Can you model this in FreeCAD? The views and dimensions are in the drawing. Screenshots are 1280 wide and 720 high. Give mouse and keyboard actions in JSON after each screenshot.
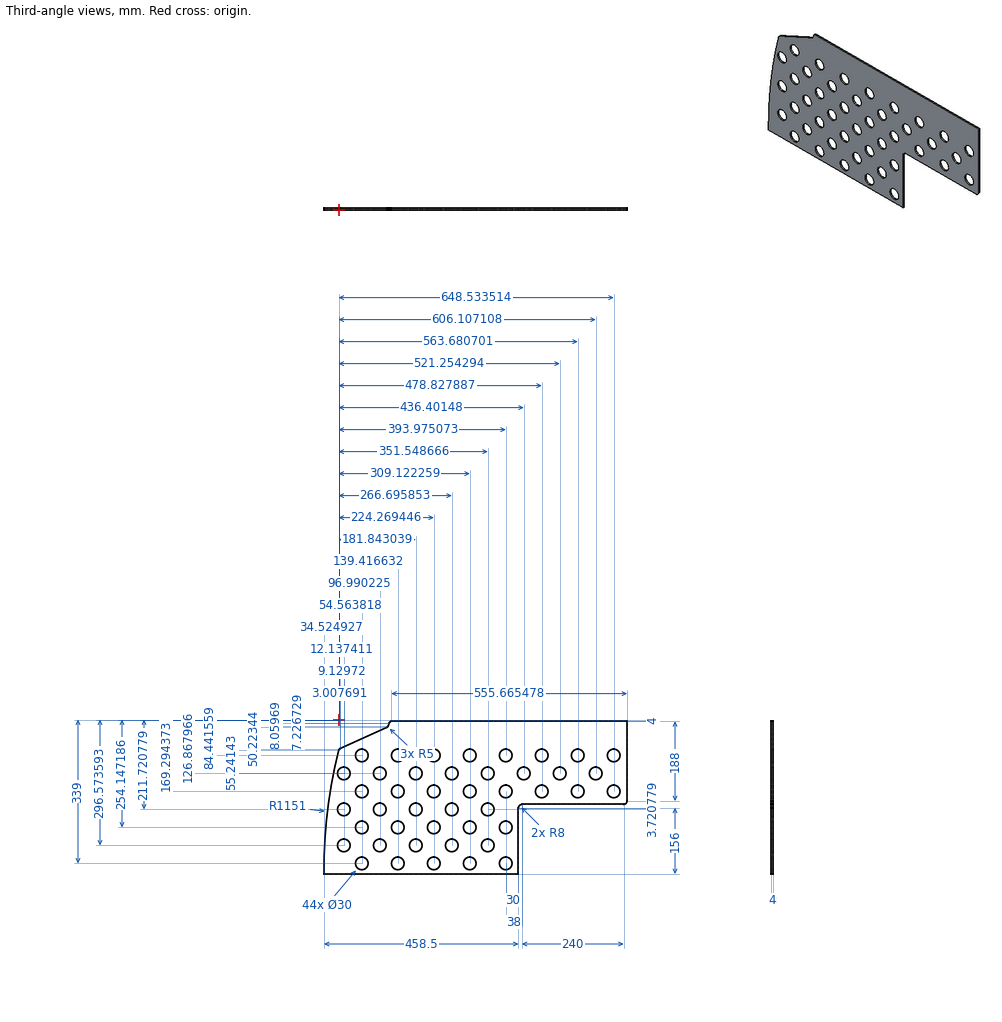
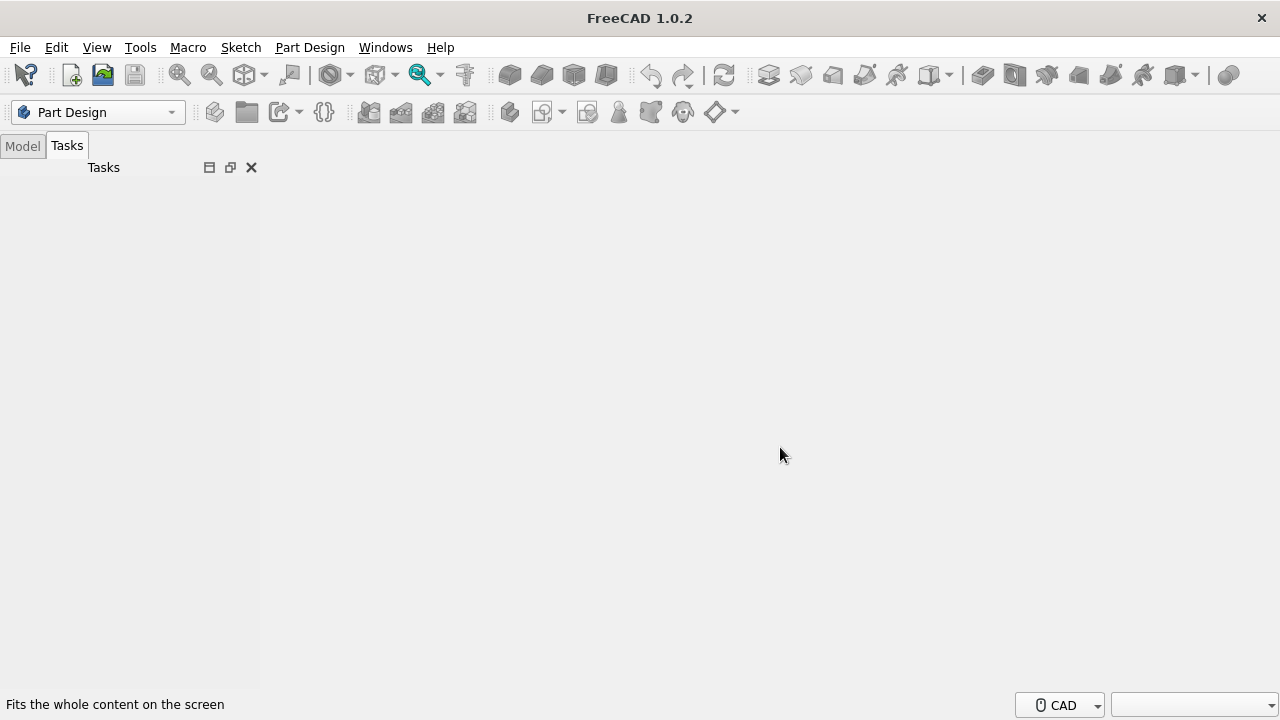
{"action": "key", "text": "ctrl+n"}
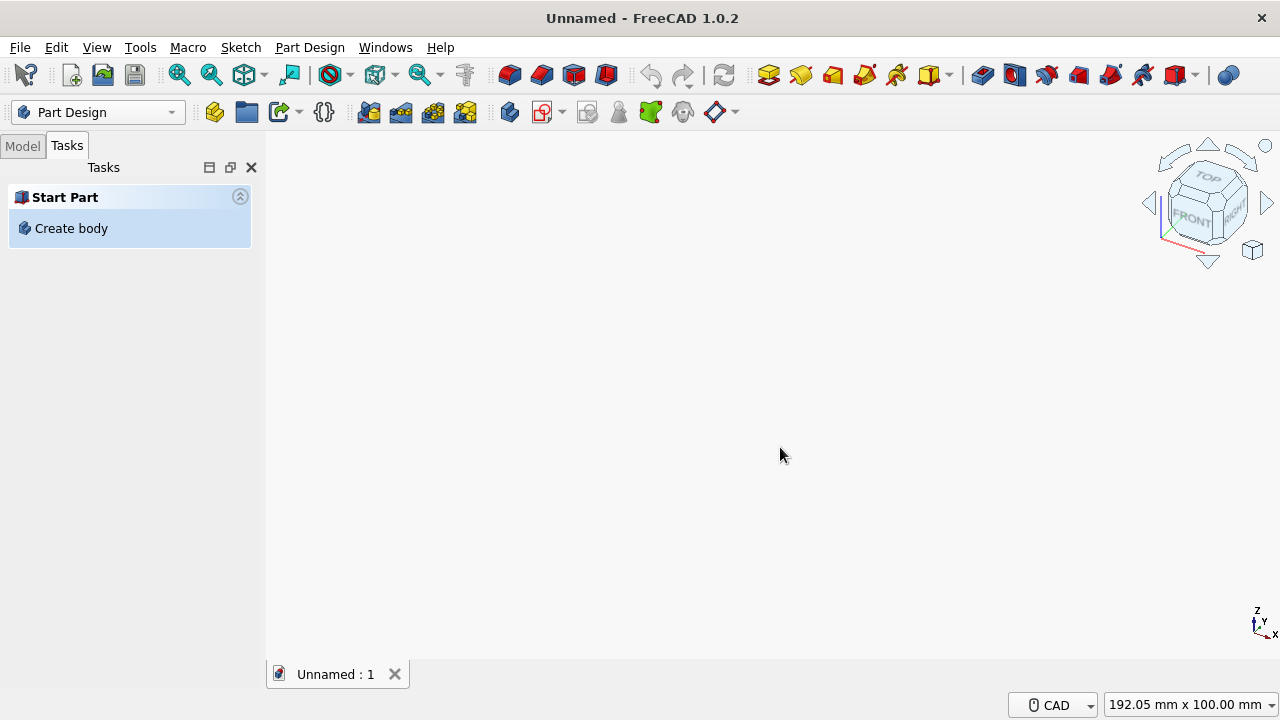
{"action": "left_click", "coordinate": [542, 112]}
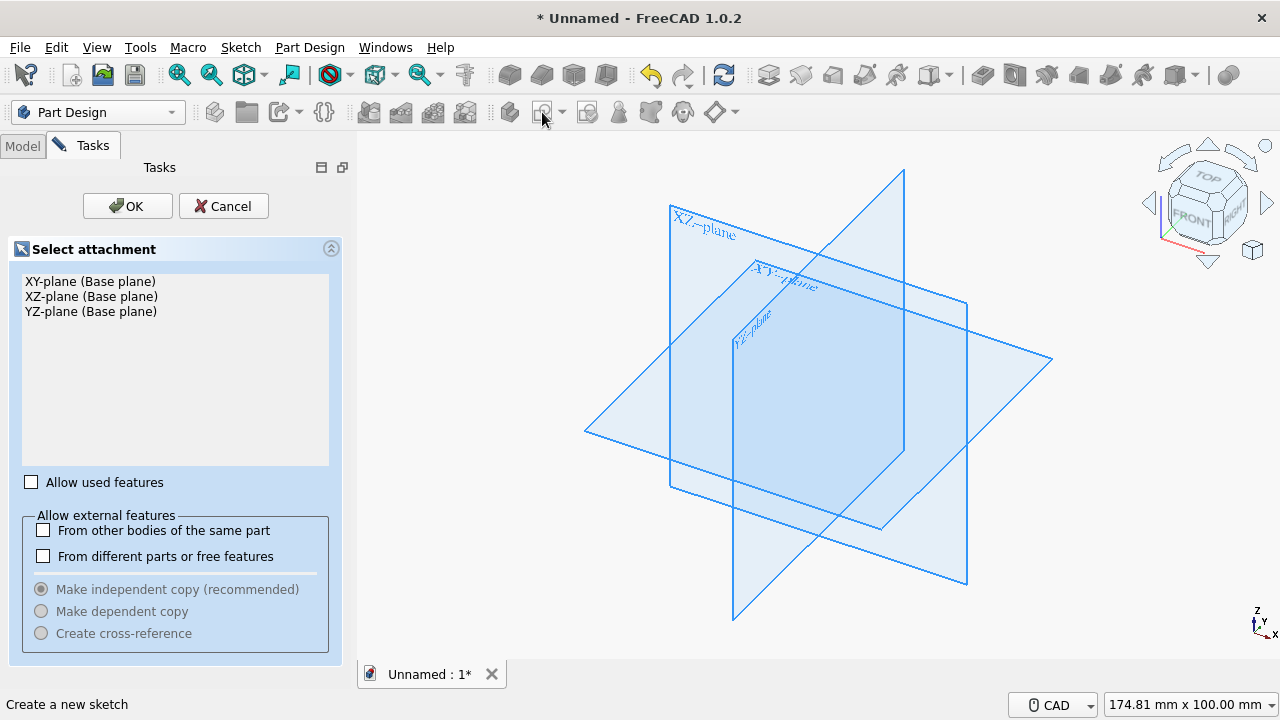
{"action": "left_click", "coordinate": [82, 296]}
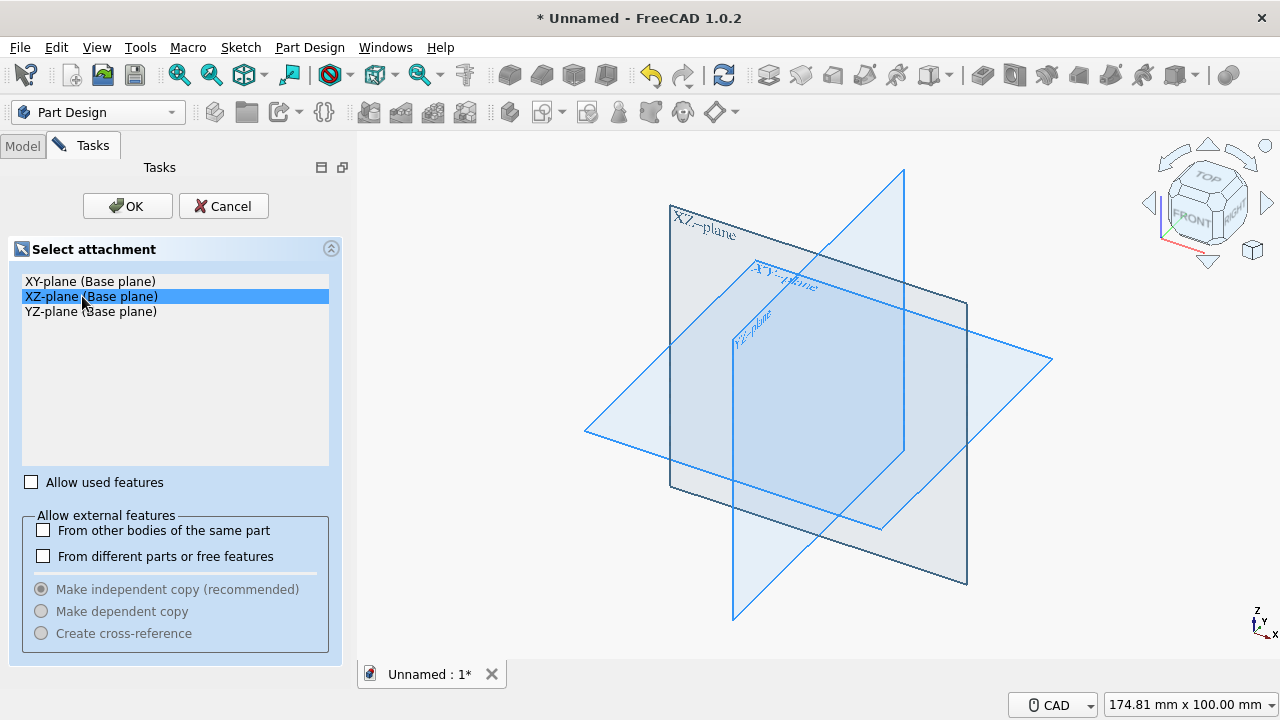
{"action": "left_click", "coordinate": [128, 206]}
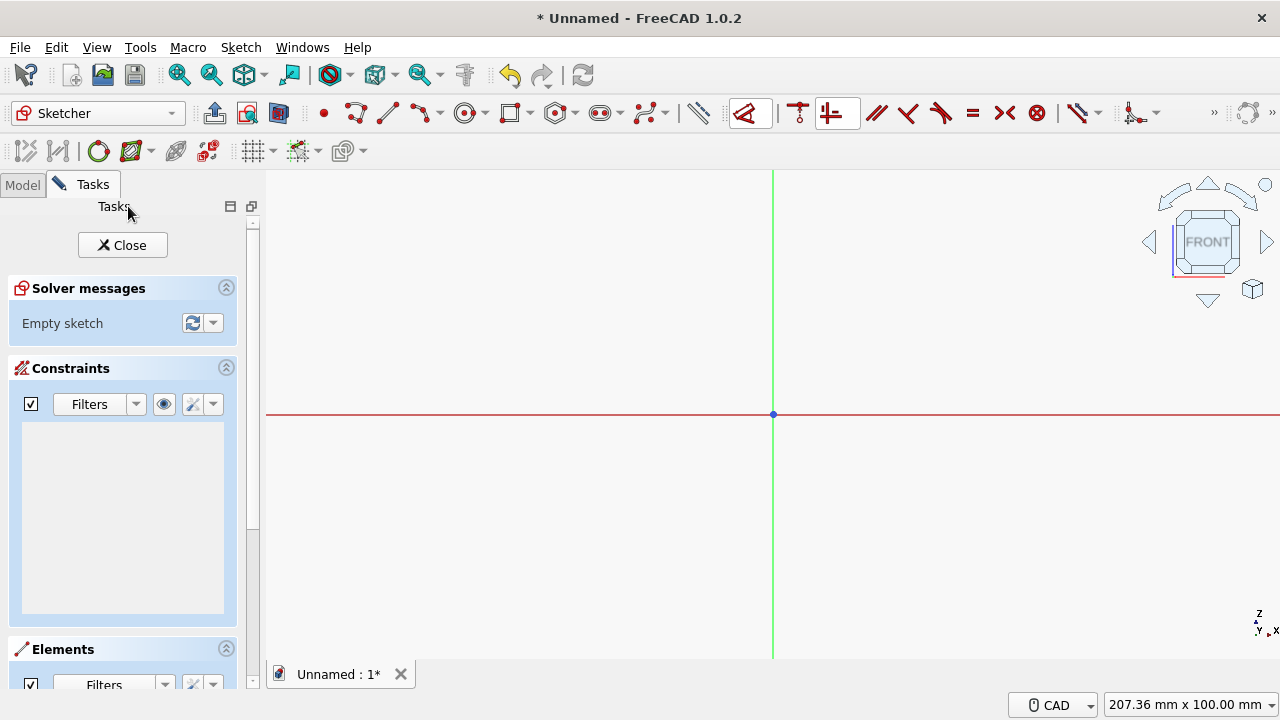
{"action": "scroll", "coordinate": [378, 238], "scroll_direction": "down", "scroll_amount": 9}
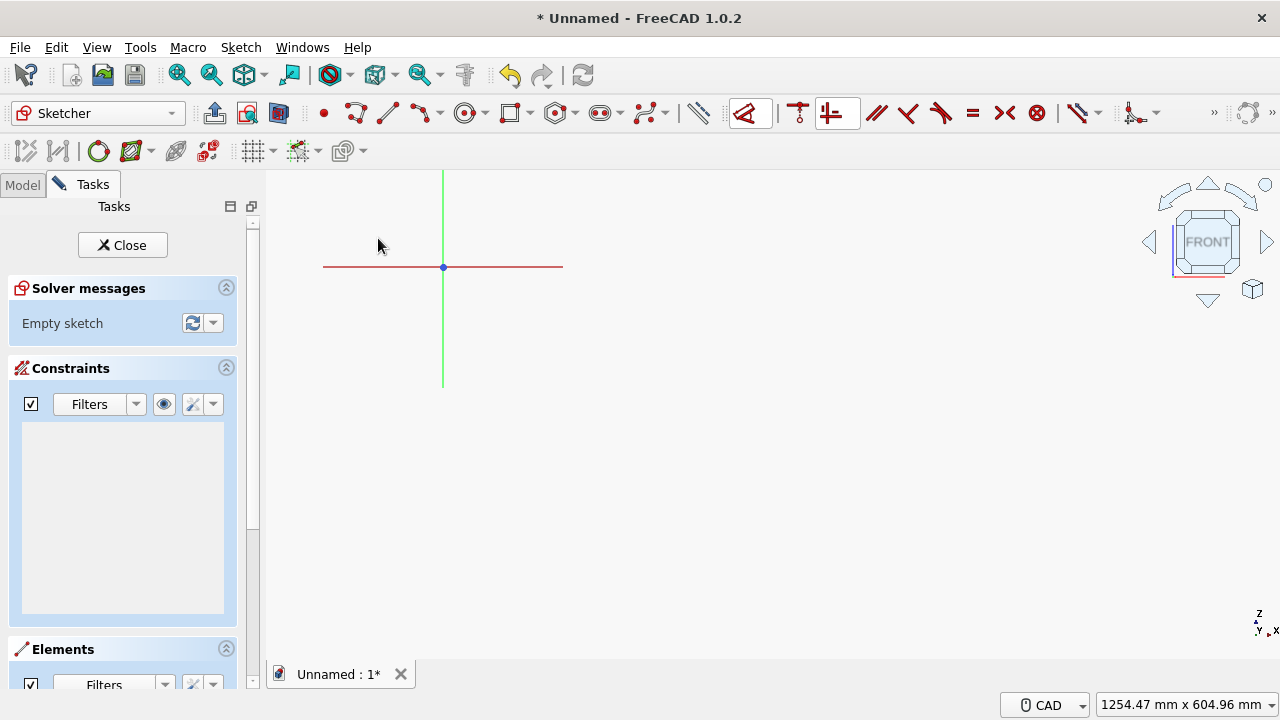
{"action": "key", "text": "g l"}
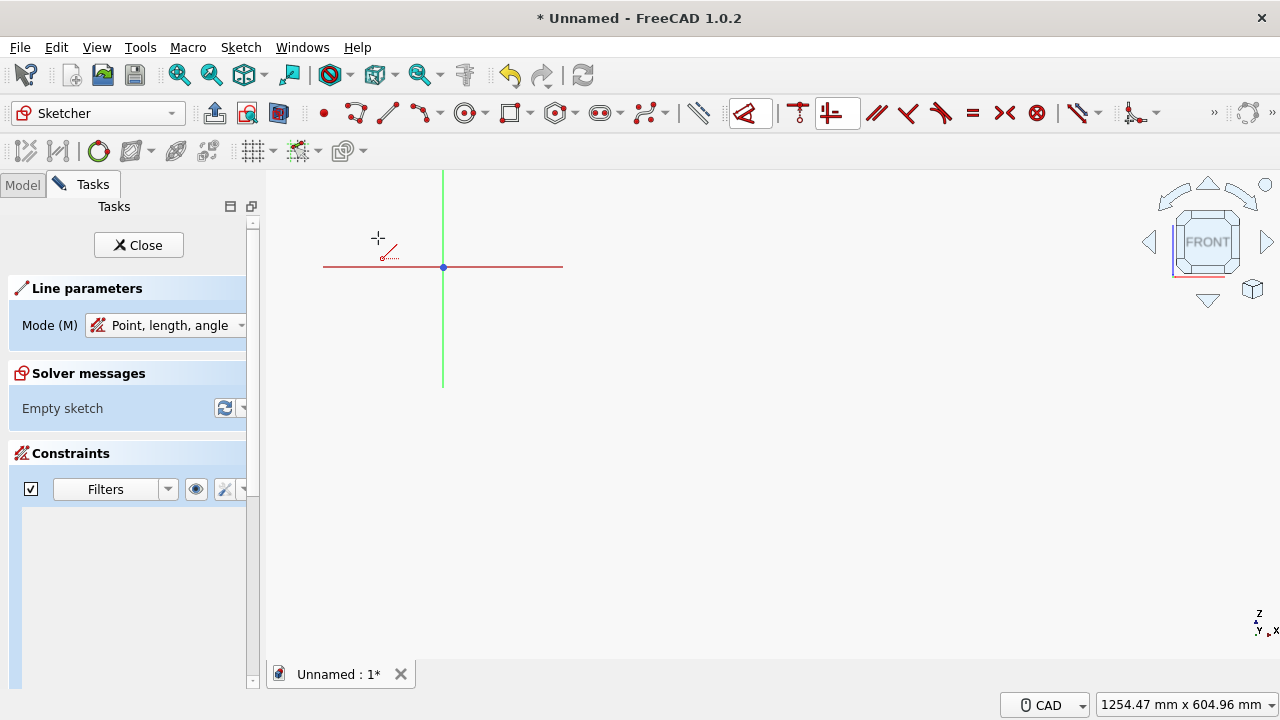
{"action": "scroll", "coordinate": [540, 273], "scroll_direction": "up", "scroll_amount": 5}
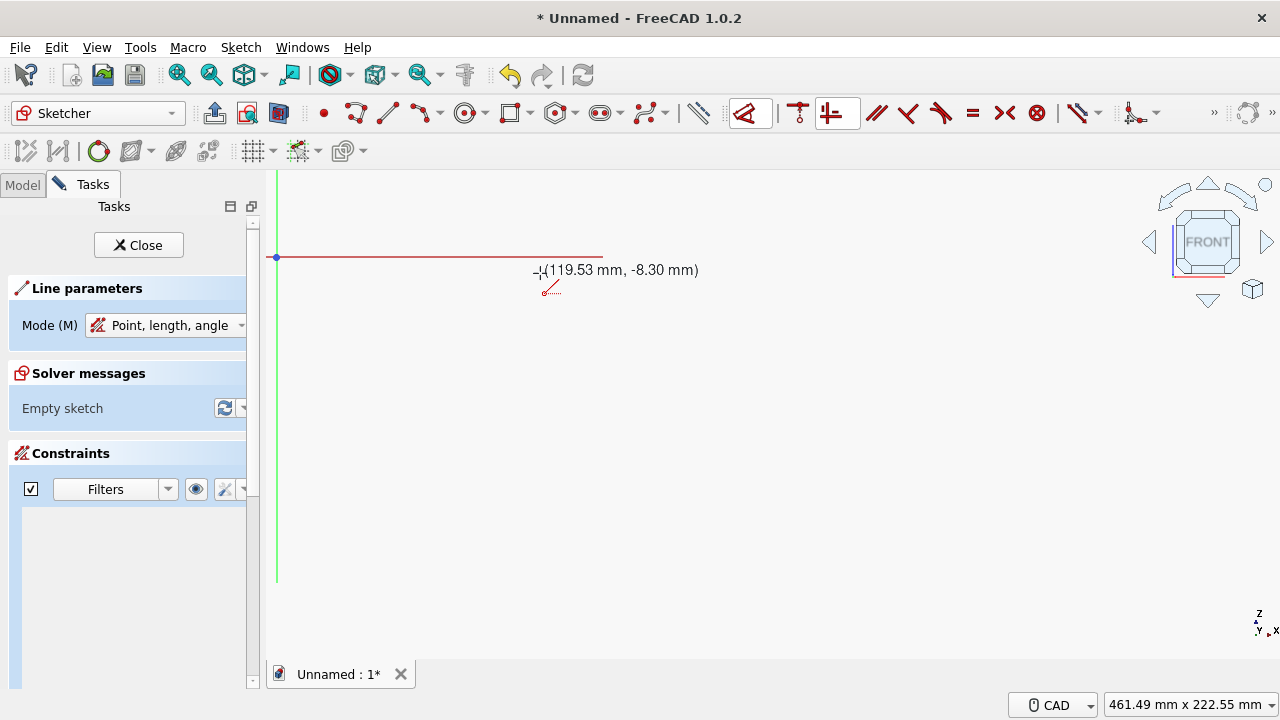
{"action": "left_click", "coordinate": [540, 273]}
{"action": "left_click", "coordinate": [533, 291]}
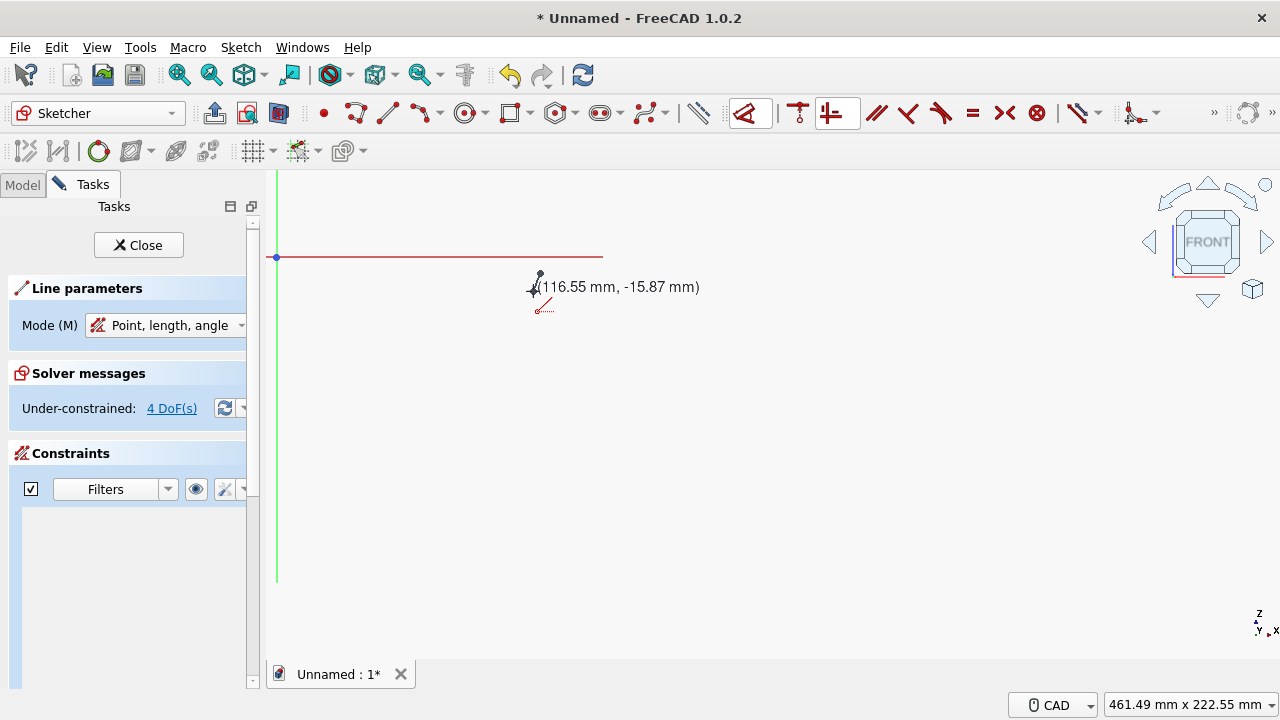
{"action": "scroll", "coordinate": [527, 297], "scroll_direction": "up", "scroll_amount": 4}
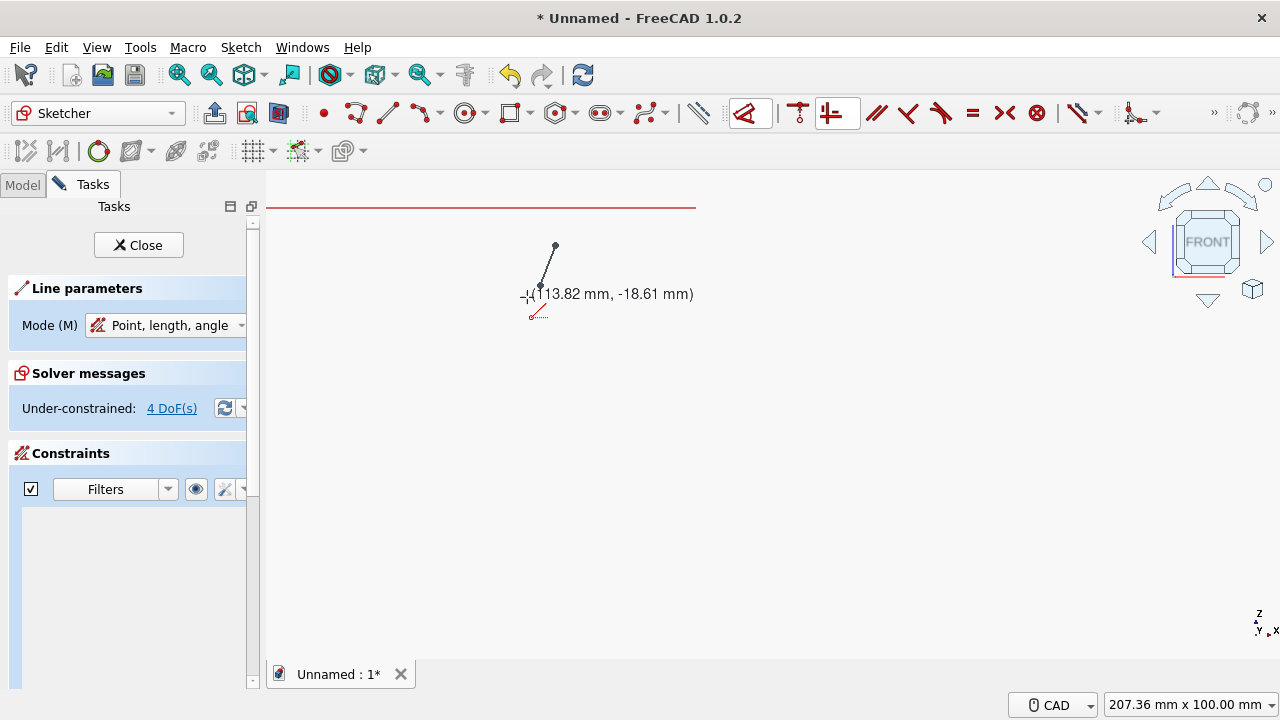
{"action": "left_click", "coordinate": [527, 296]}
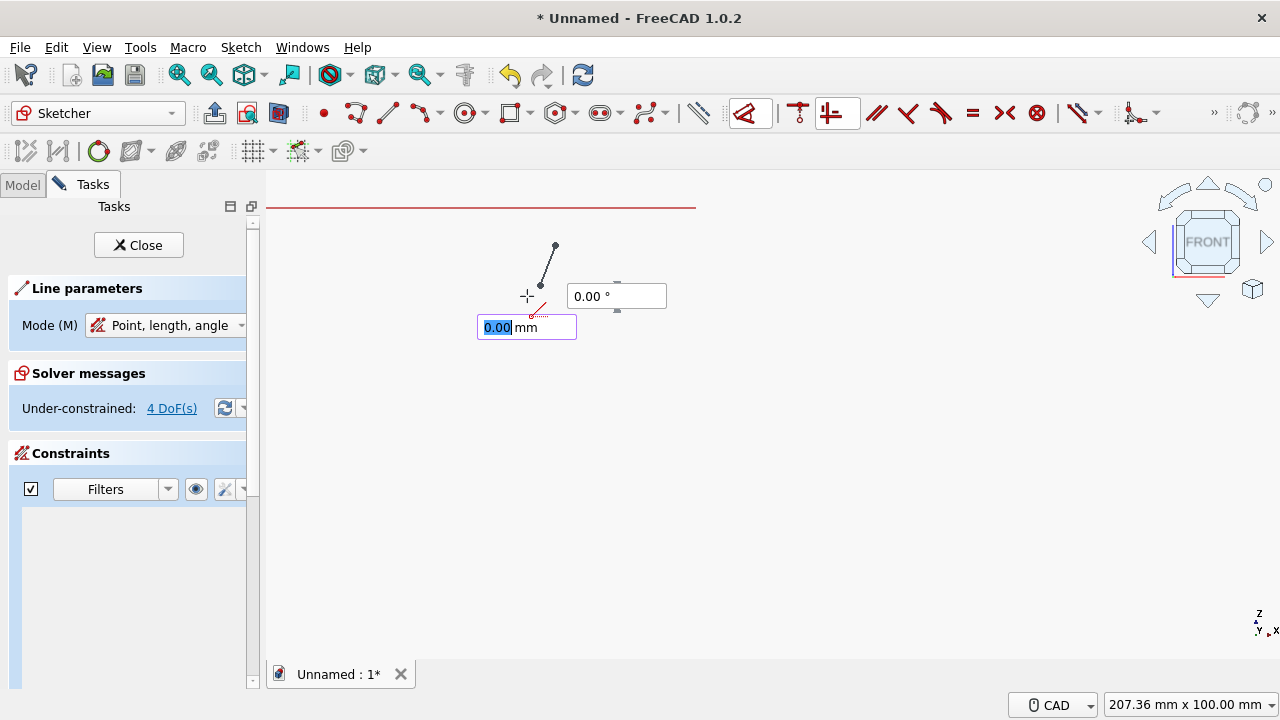
{"action": "scroll", "coordinate": [537, 279], "scroll_direction": "down", "scroll_amount": 9}